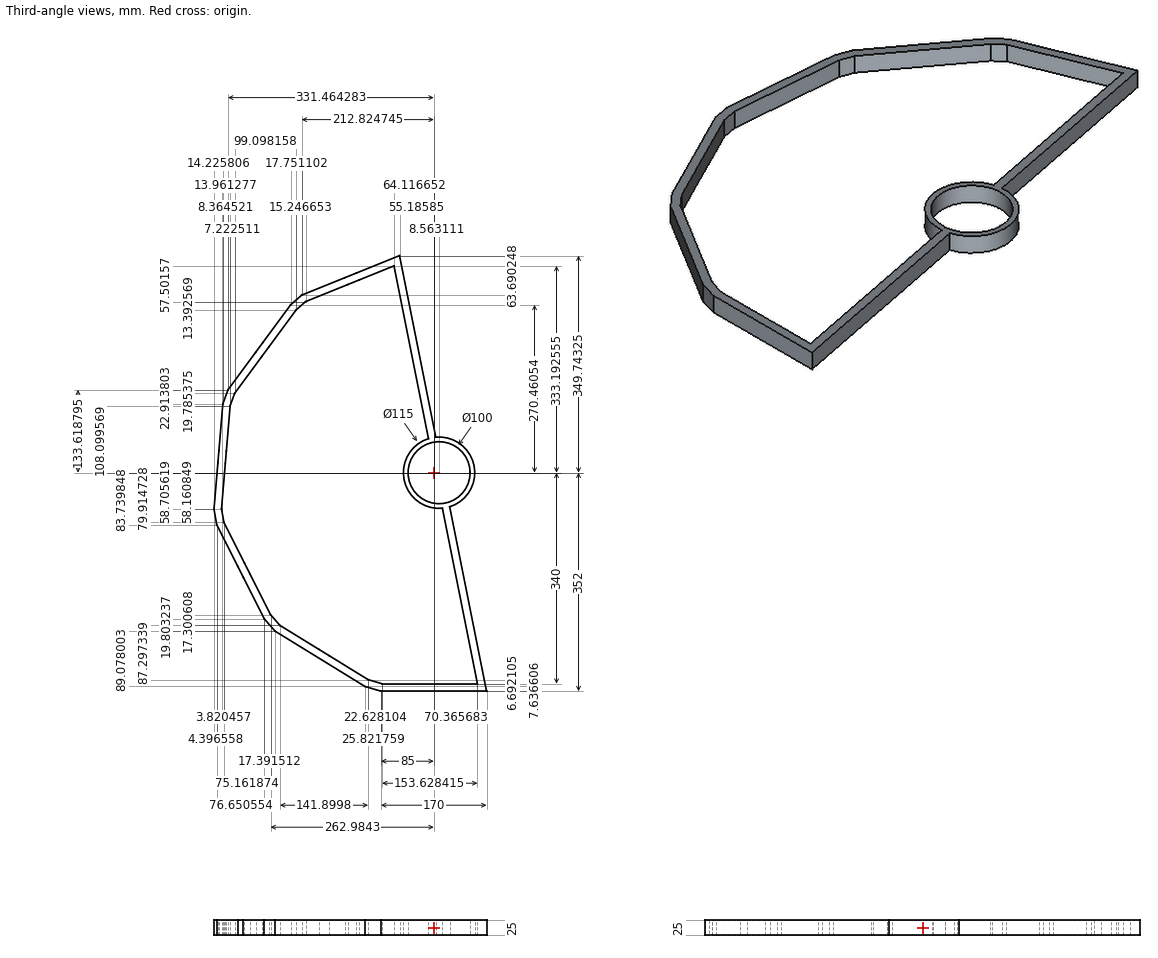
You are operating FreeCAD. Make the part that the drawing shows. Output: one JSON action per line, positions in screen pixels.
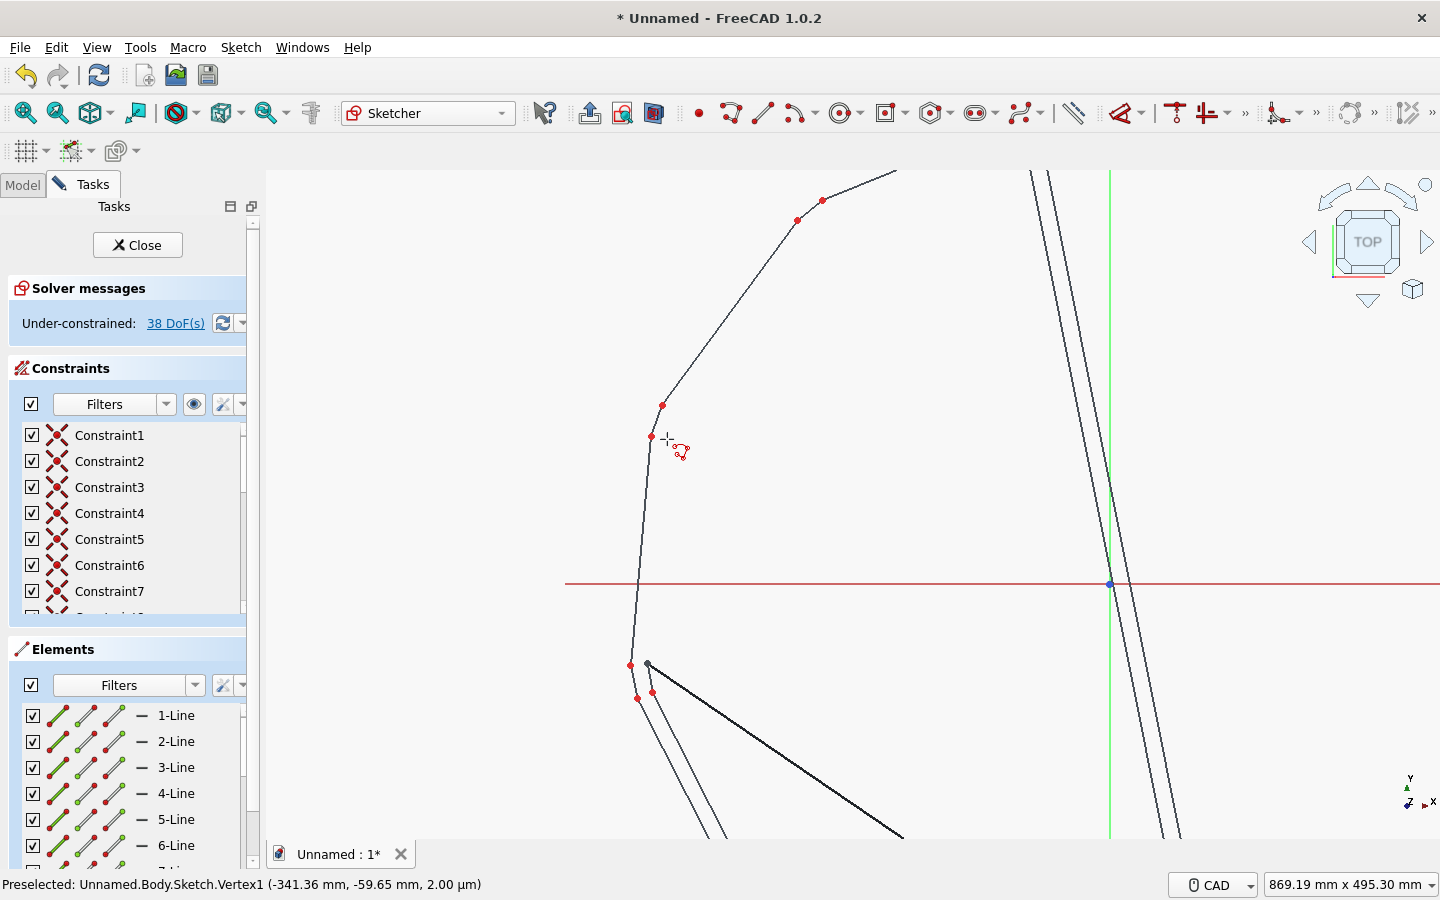
{"action": "left_click", "coordinate": [667, 438]}
{"action": "left_click", "coordinate": [677, 412]}
{"action": "left_click", "coordinate": [810, 230]}
{"action": "left_click", "coordinate": [831, 212]}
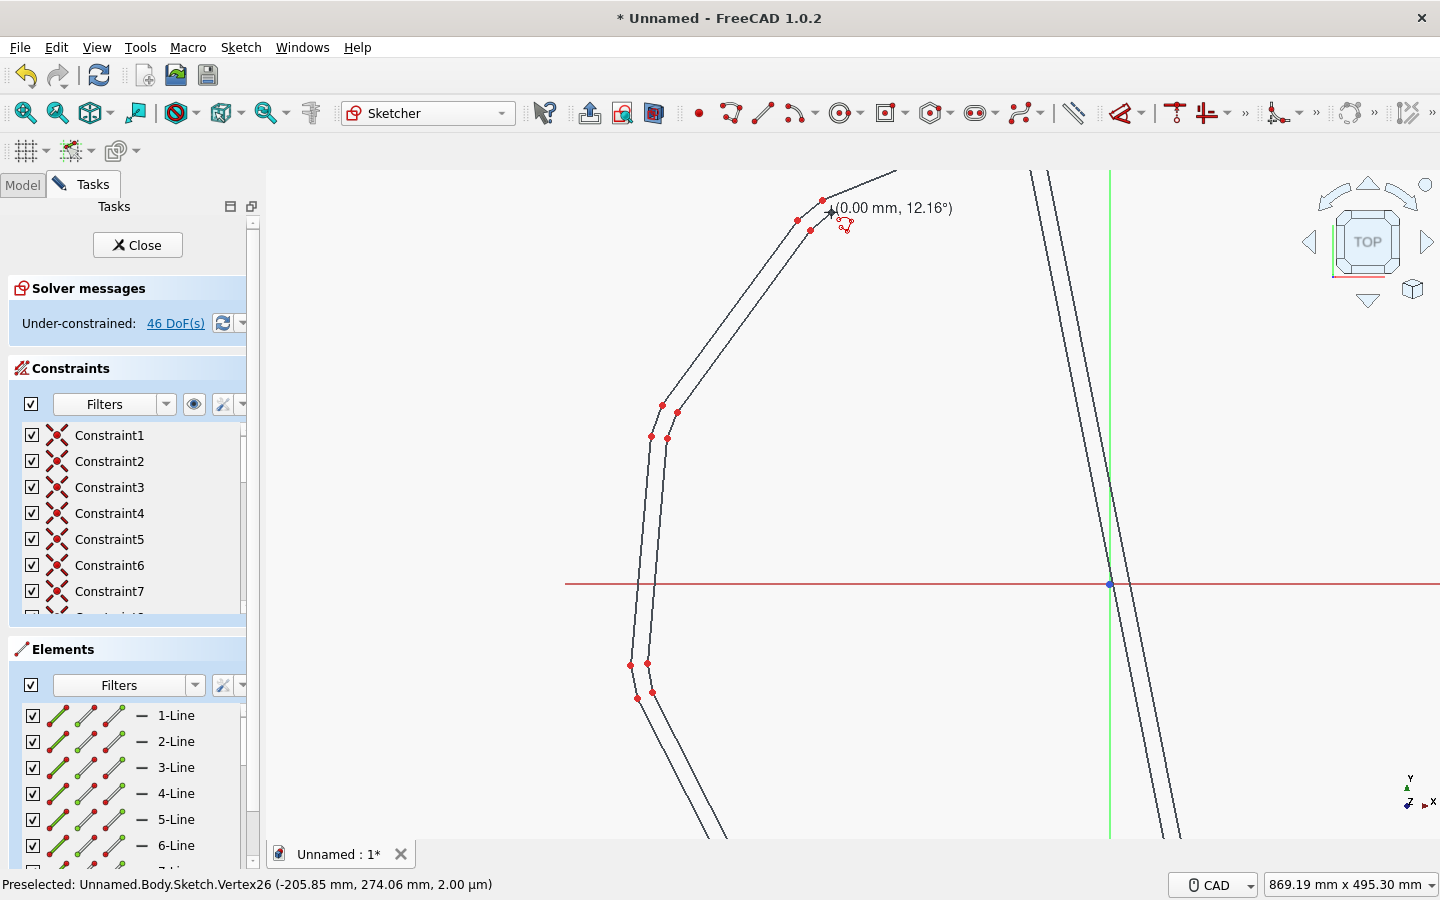
{"action": "scroll", "coordinate": [667, 438], "scroll_direction": "down", "scroll_amount": 4}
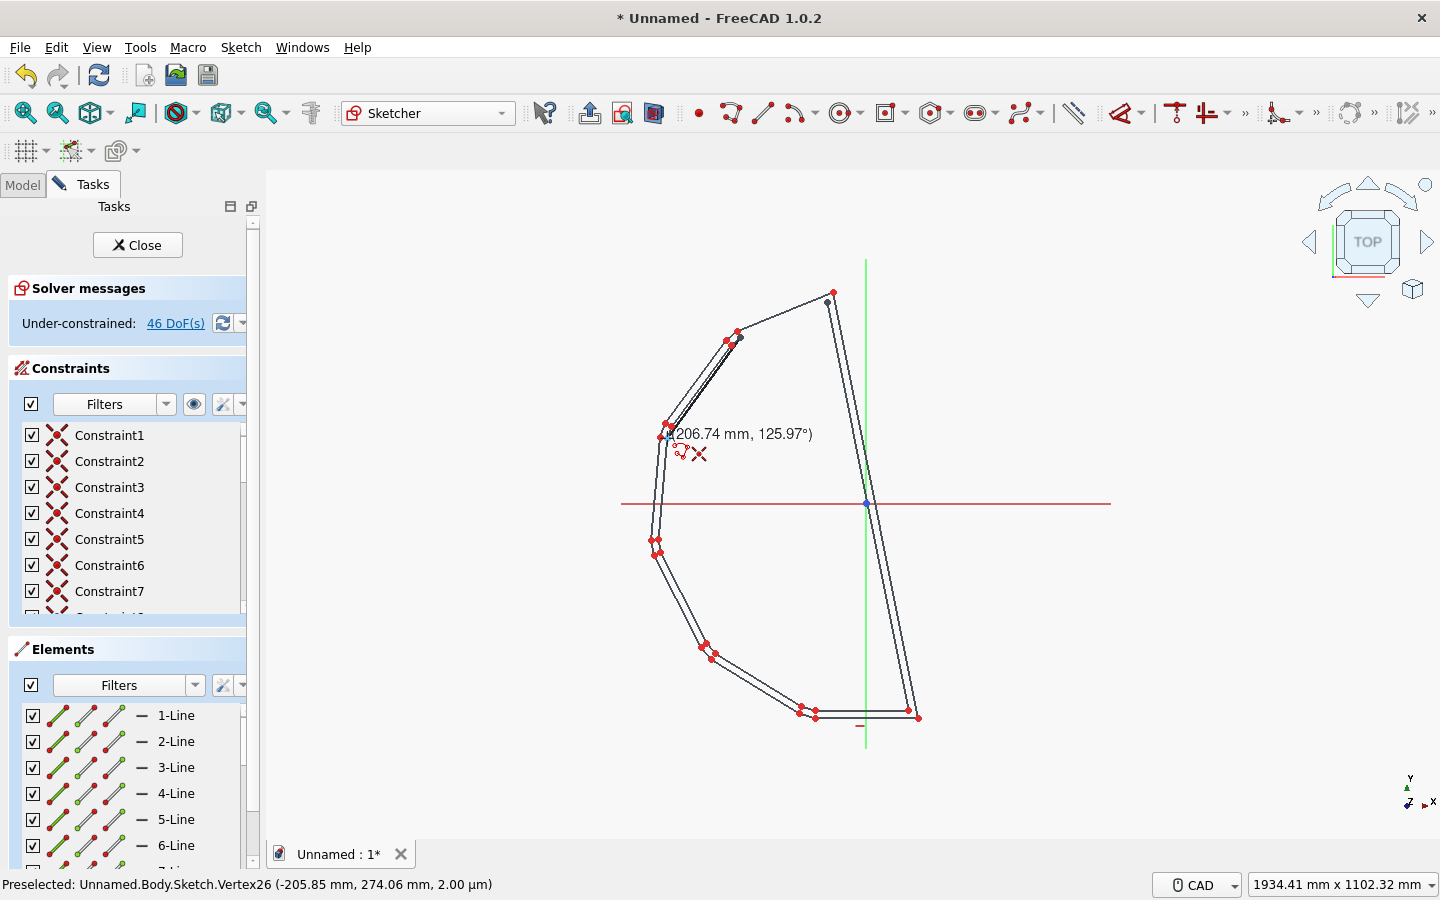
{"action": "scroll", "coordinate": [827, 302], "scroll_direction": "up", "scroll_amount": 4}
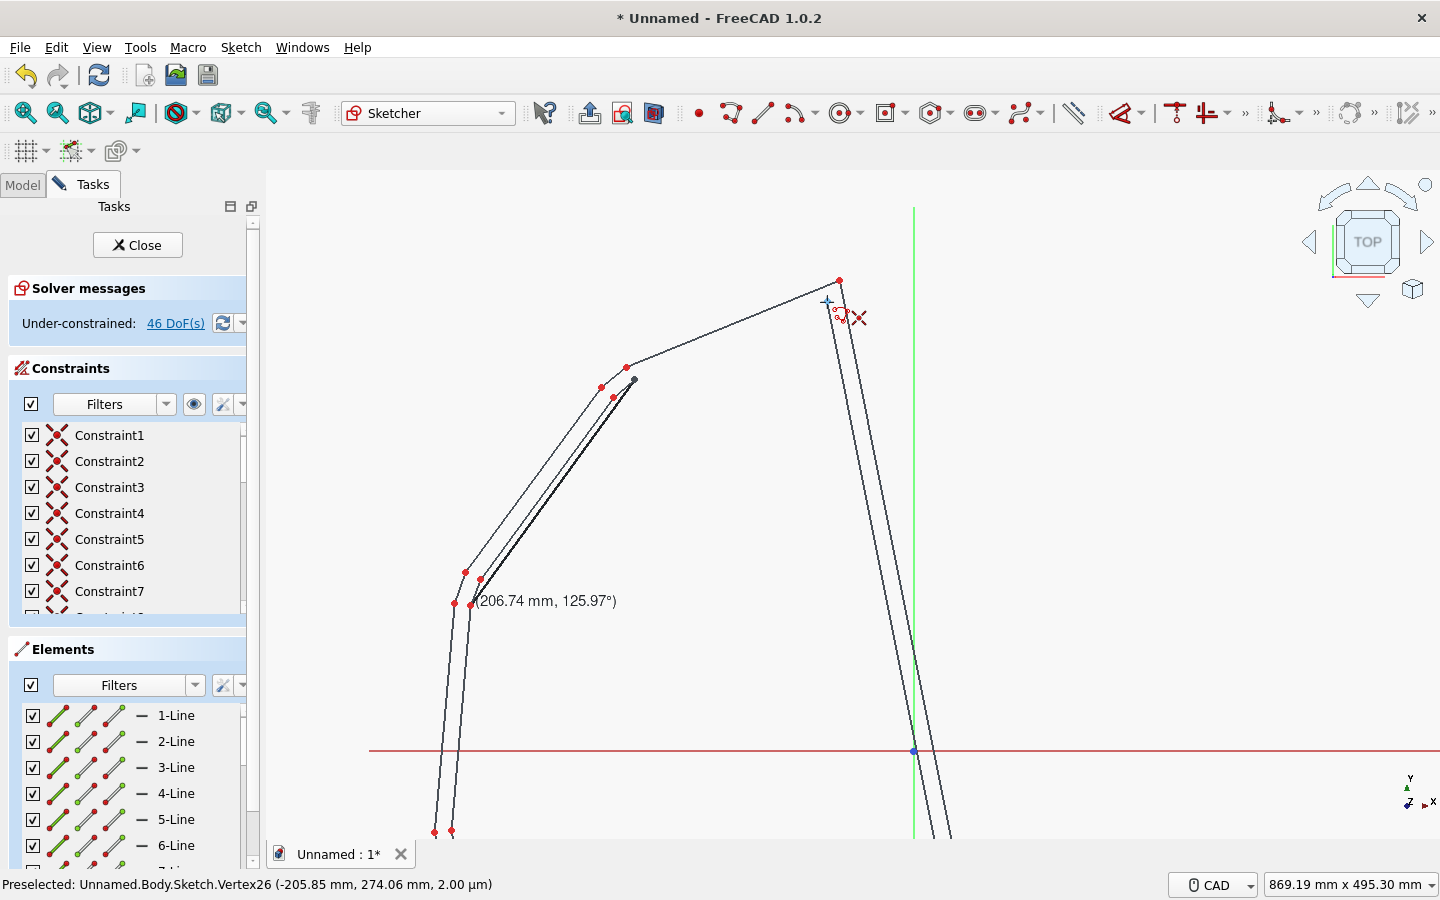
{"action": "left_click", "coordinate": [827, 302]}
{"action": "key", "text": "Escape"}
{"action": "key", "text": "Escape"}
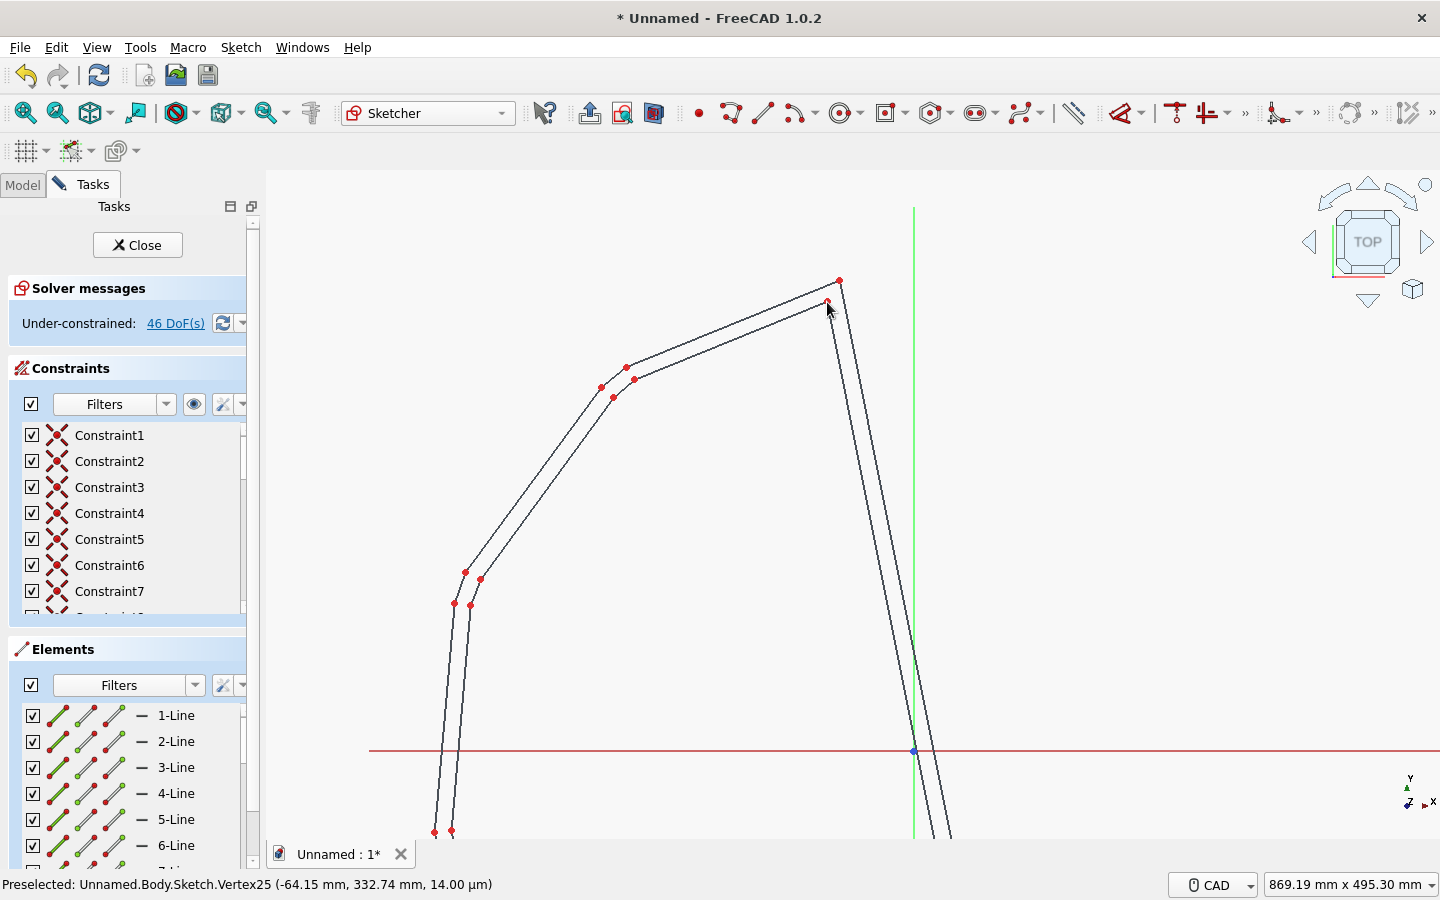
{"action": "left_click", "coordinate": [1120, 114]}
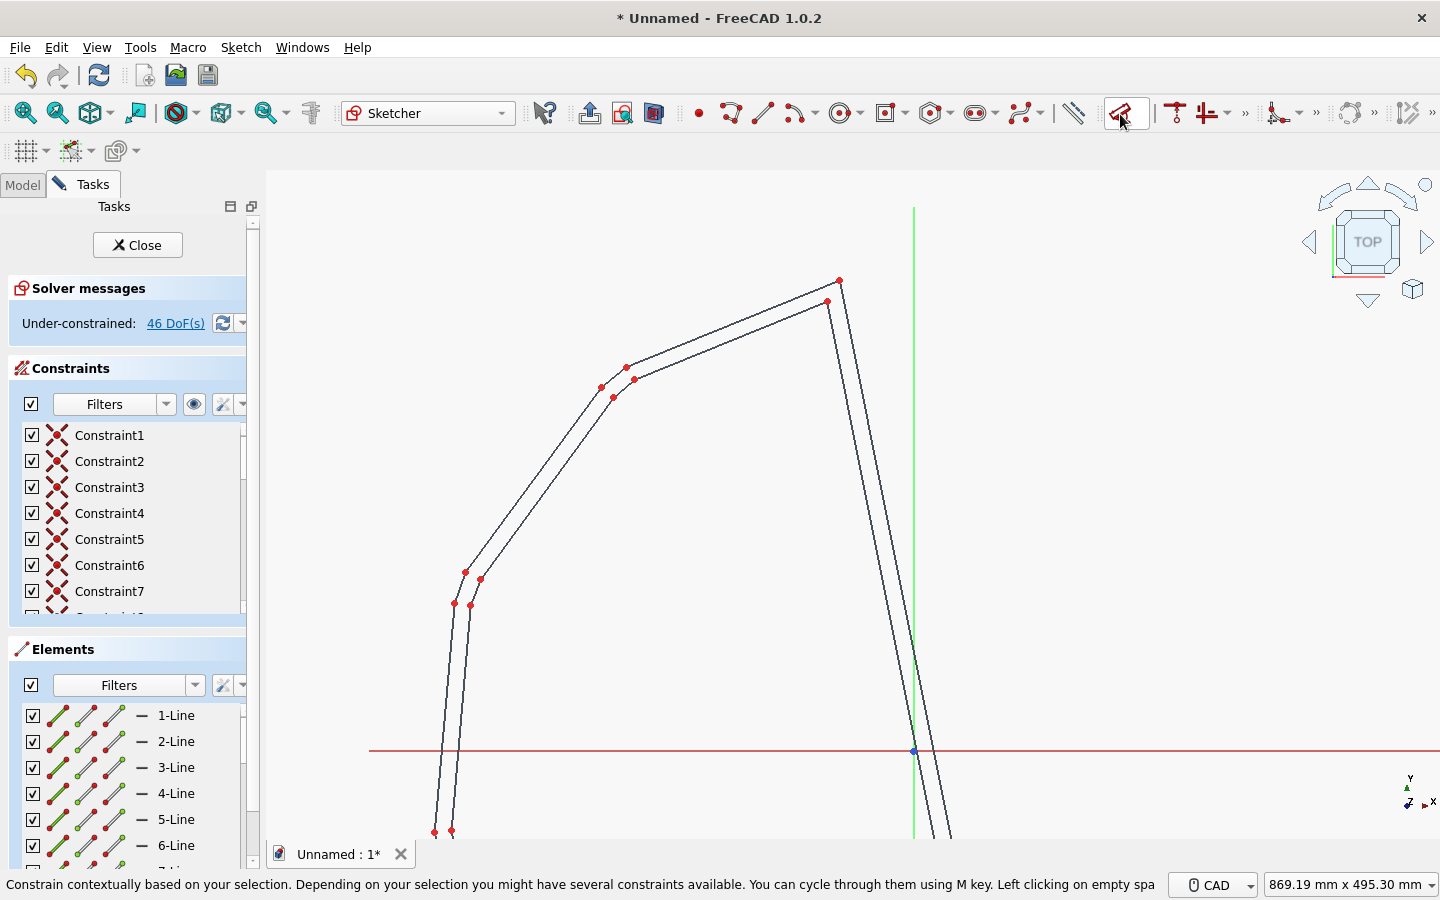
{"action": "scroll", "coordinate": [827, 302], "scroll_direction": "down", "scroll_amount": 4}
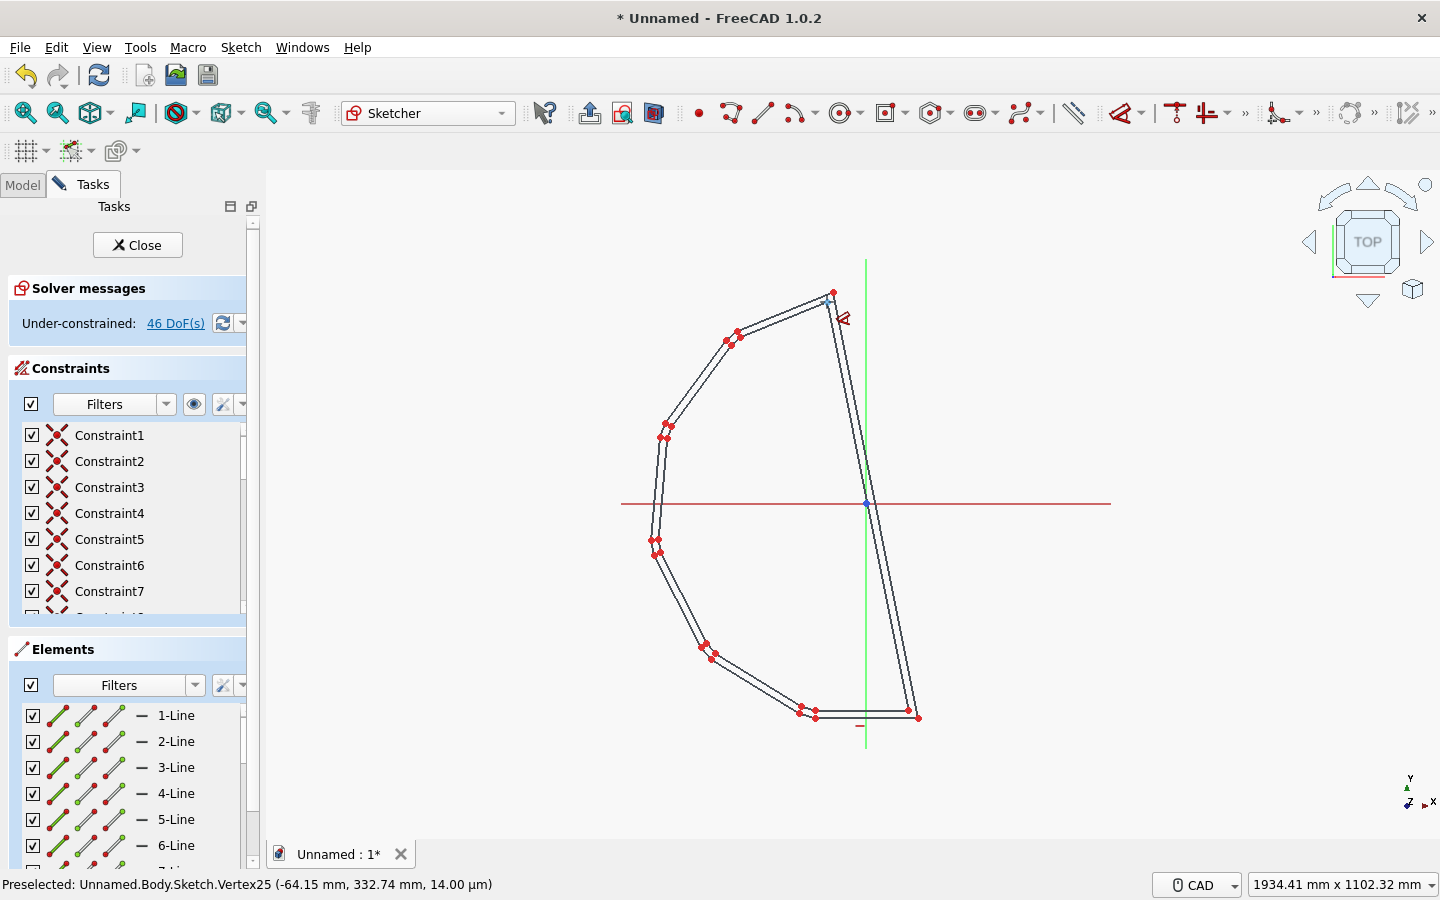
{"action": "scroll", "coordinate": [846, 718], "scroll_direction": "up", "scroll_amount": 4}